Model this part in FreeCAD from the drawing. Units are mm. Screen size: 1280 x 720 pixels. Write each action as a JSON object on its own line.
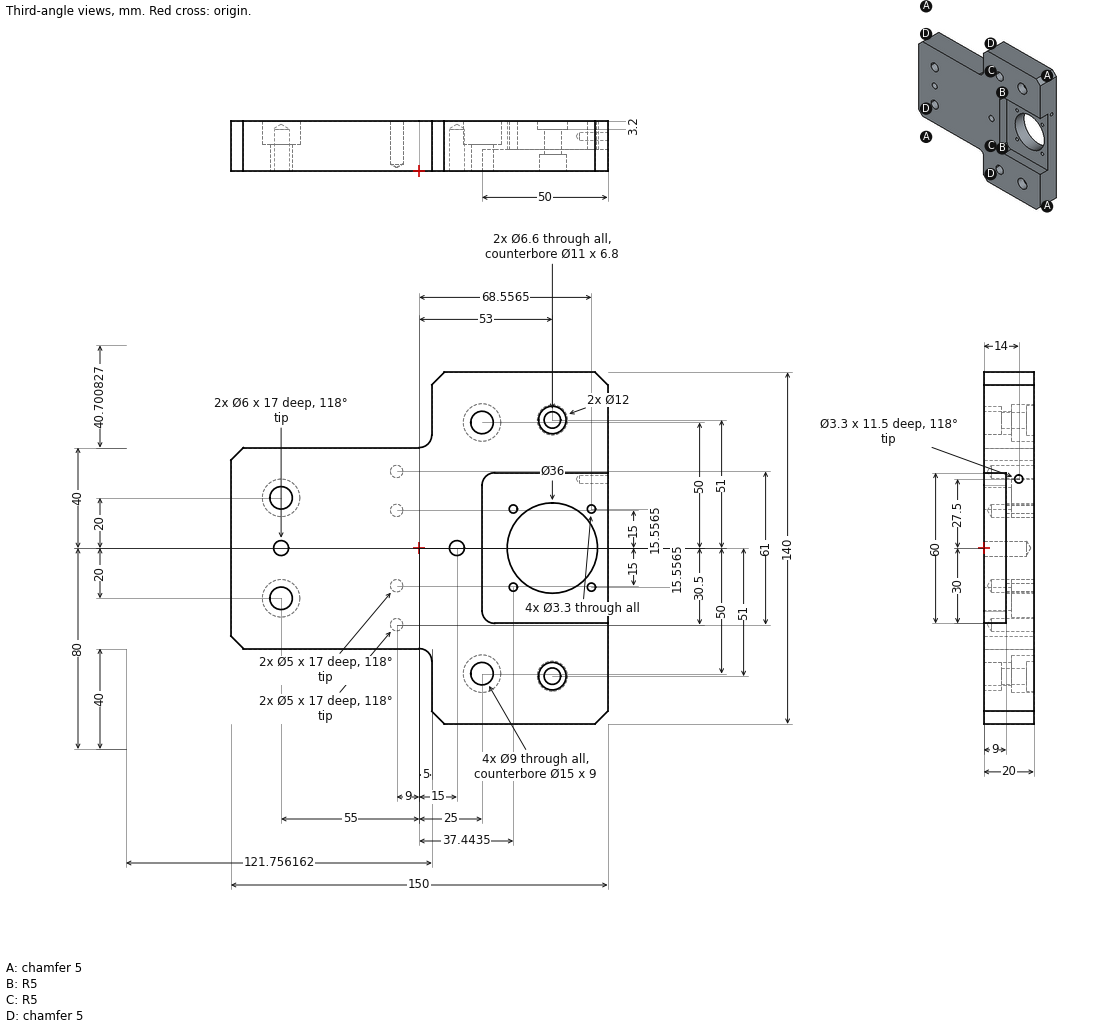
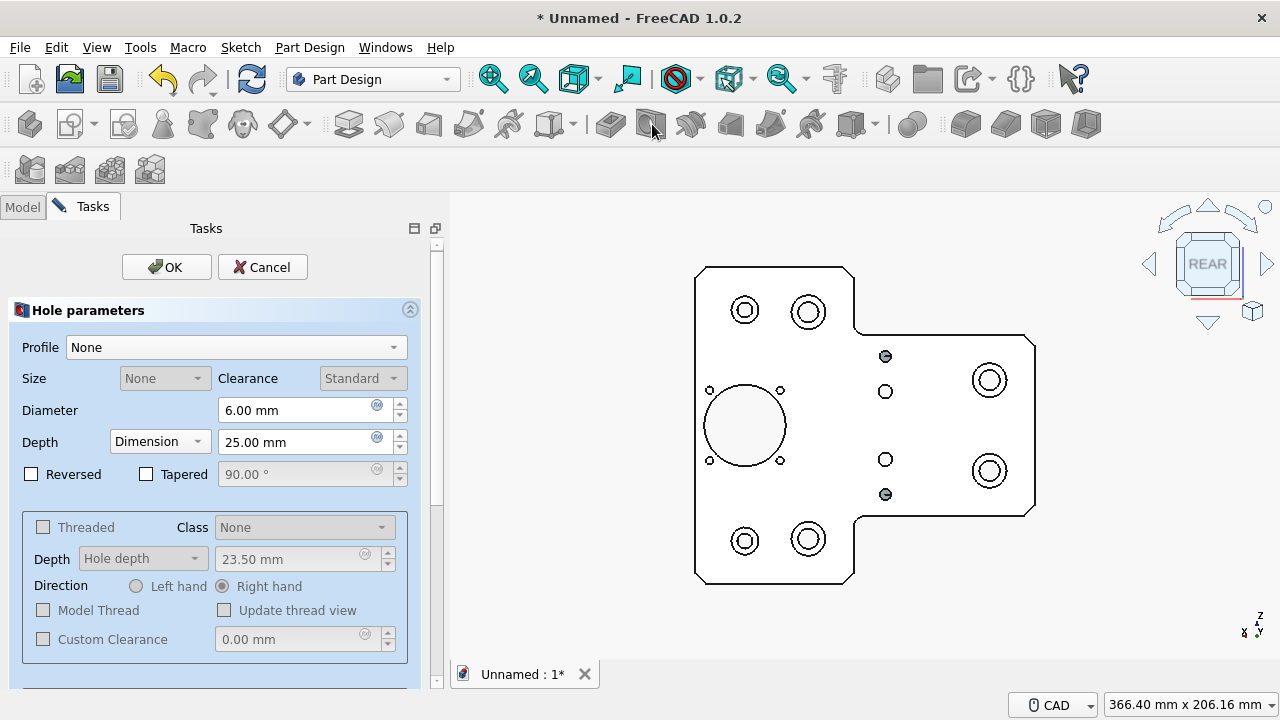
{"action": "triple_click", "coordinate": [305, 410]}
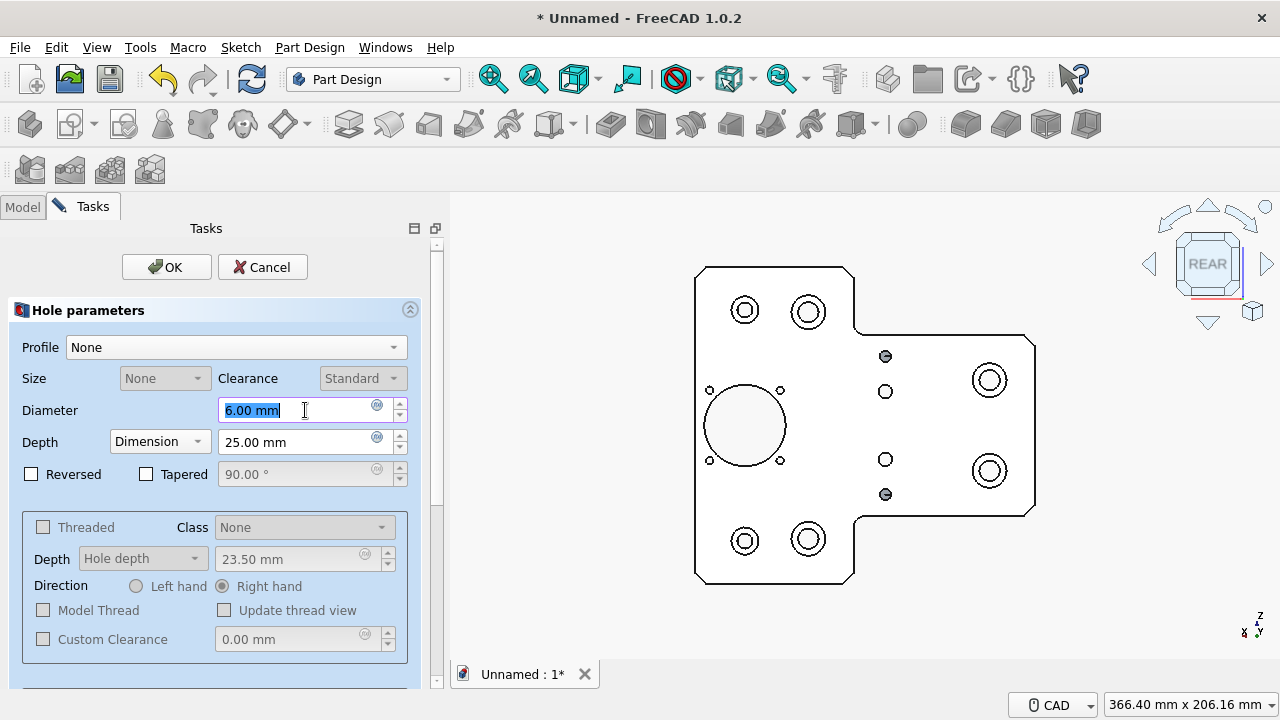
{"action": "type", "text": "5"}
{"action": "key", "text": "Tab"}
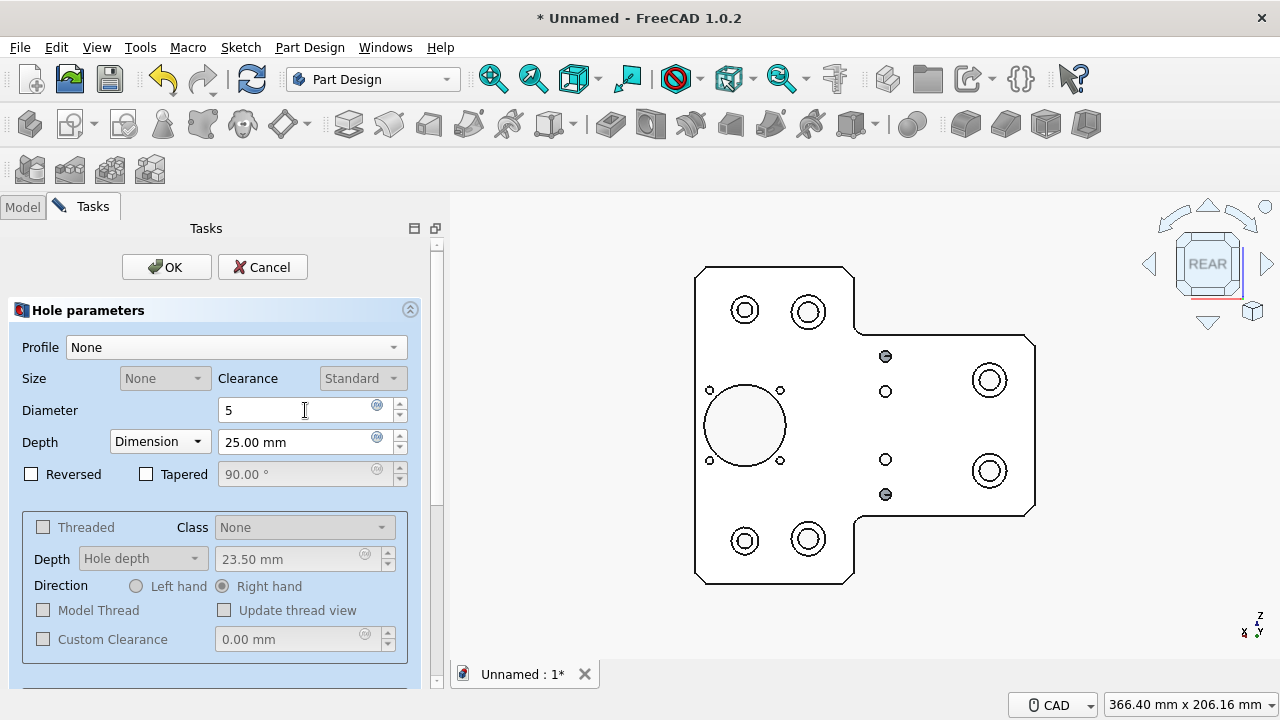
{"action": "triple_click", "coordinate": [305, 442]}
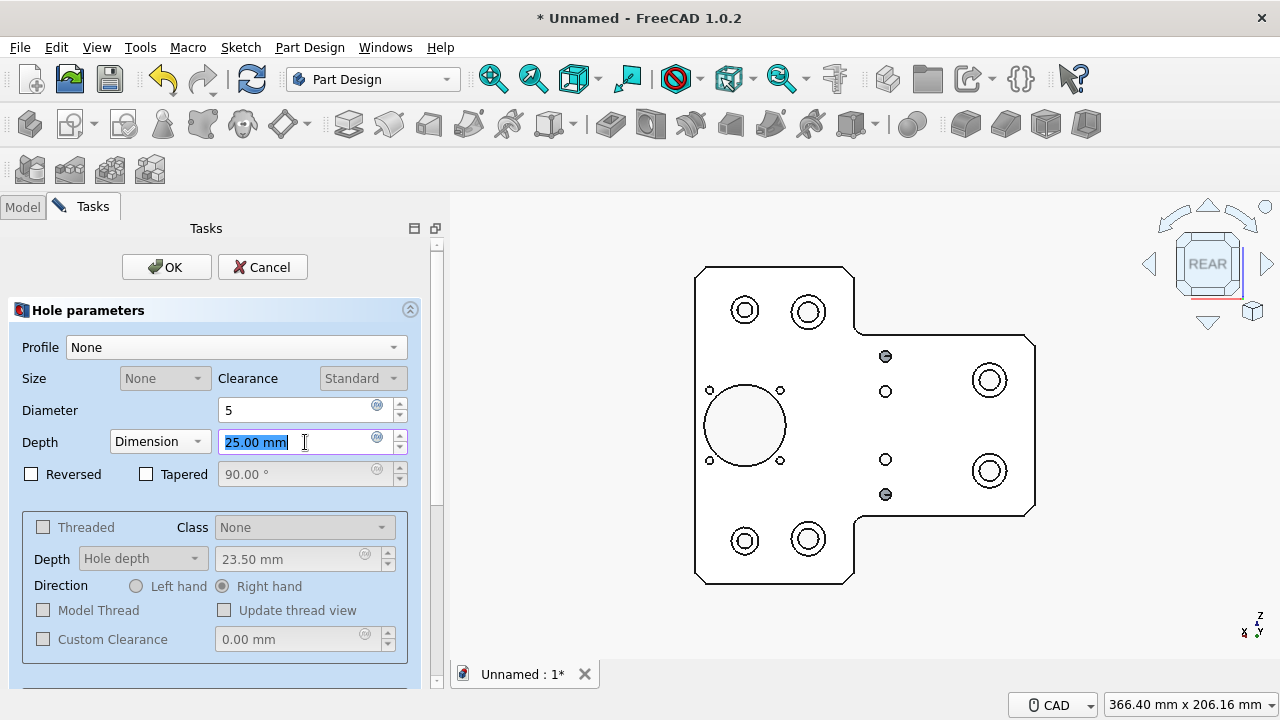
{"action": "type", "text": "17"}
{"action": "key", "text": "Tab"}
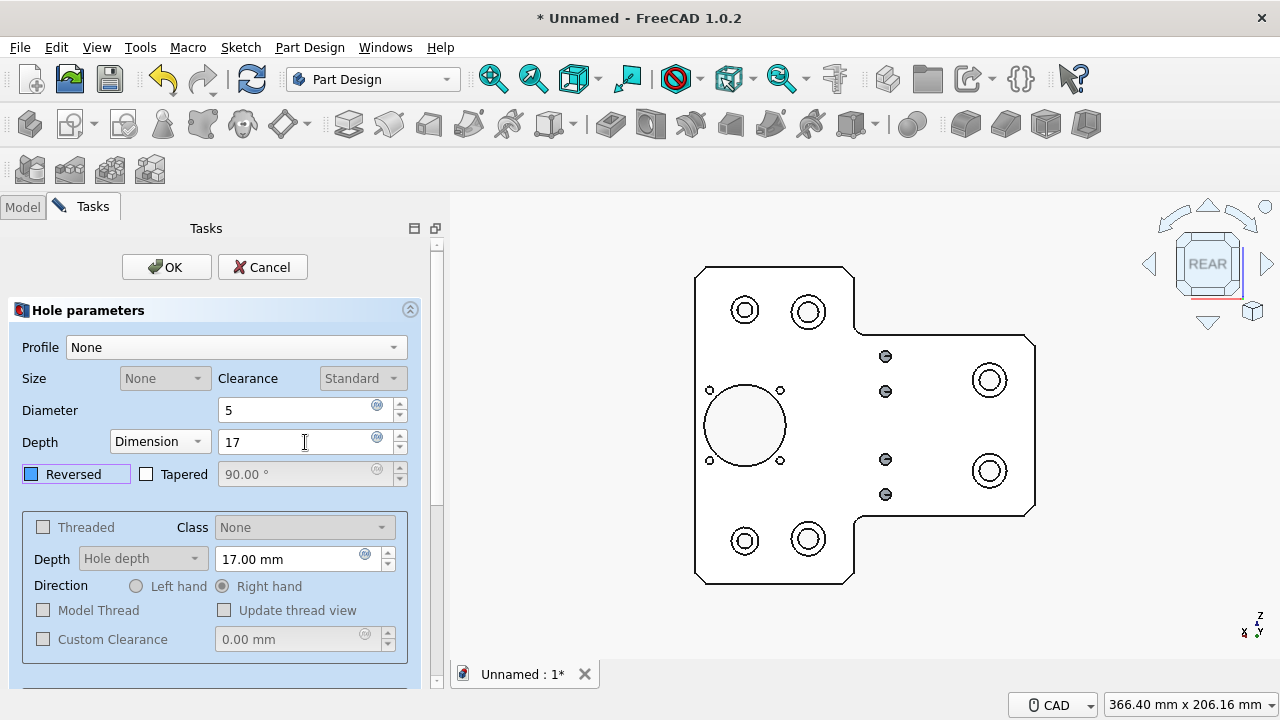
{"action": "left_click", "coordinate": [167, 267]}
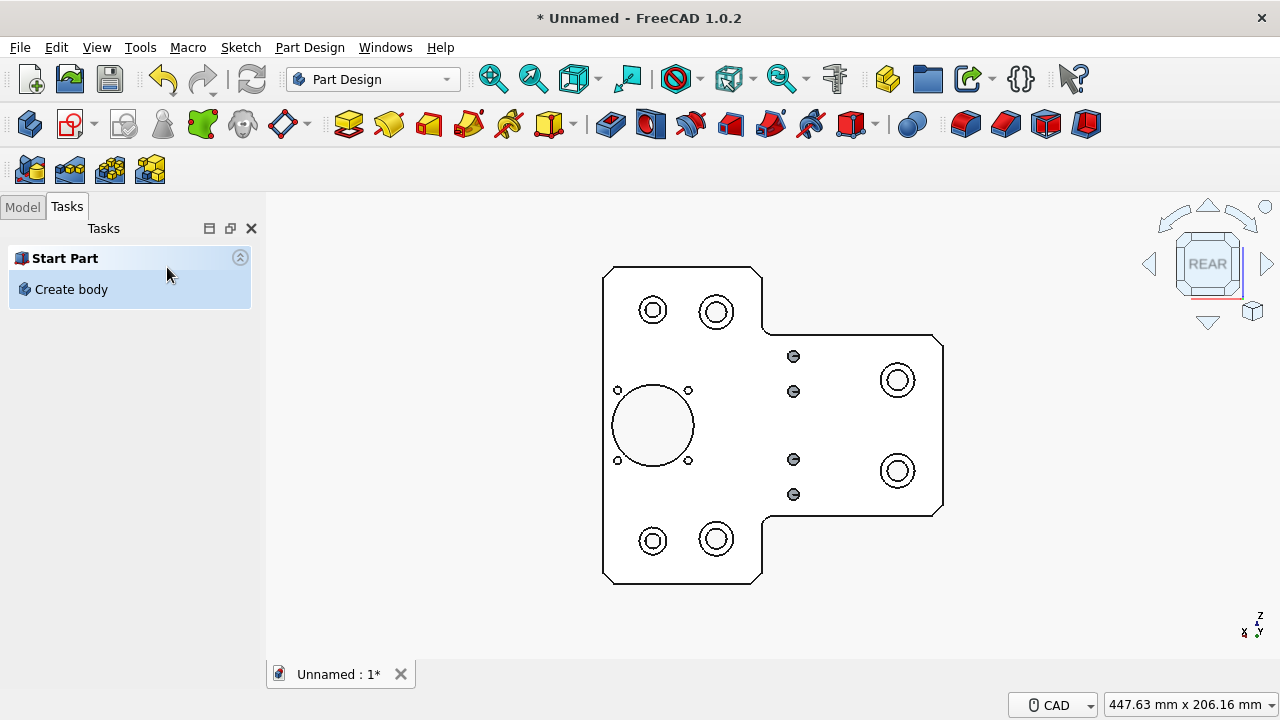
{"action": "key", "text": "0"}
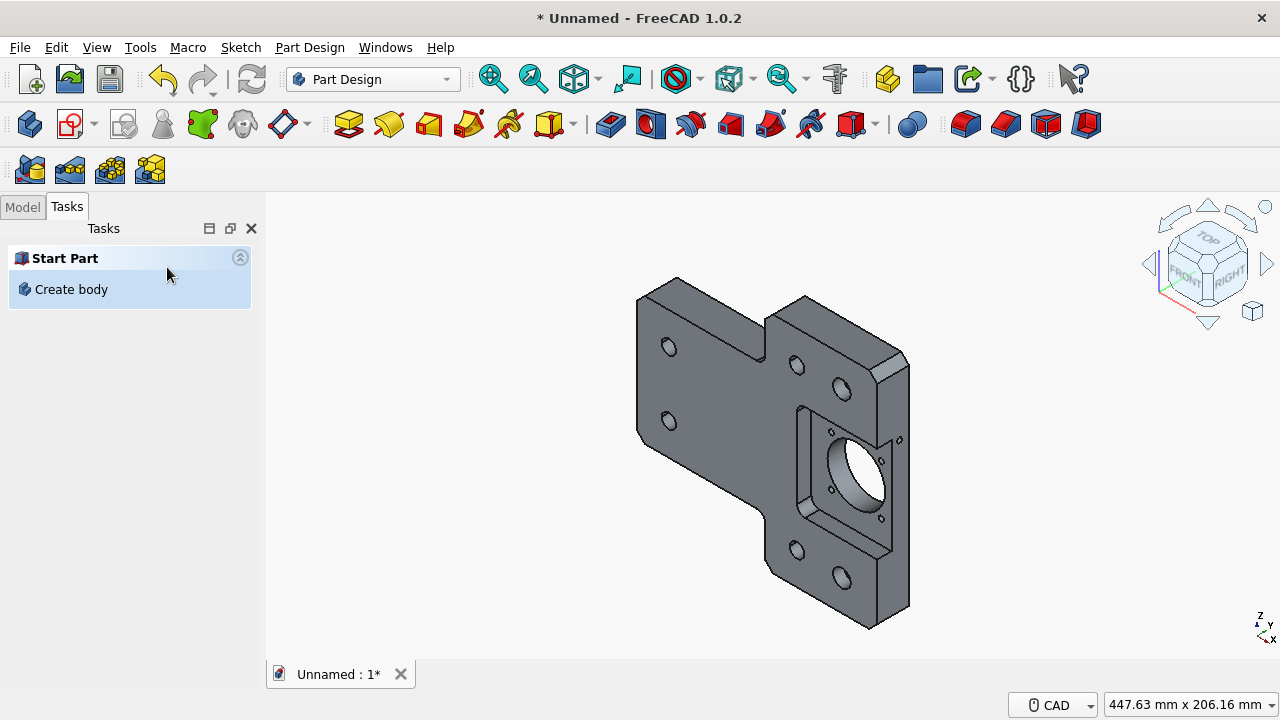
{"action": "left_click", "coordinate": [723, 414]}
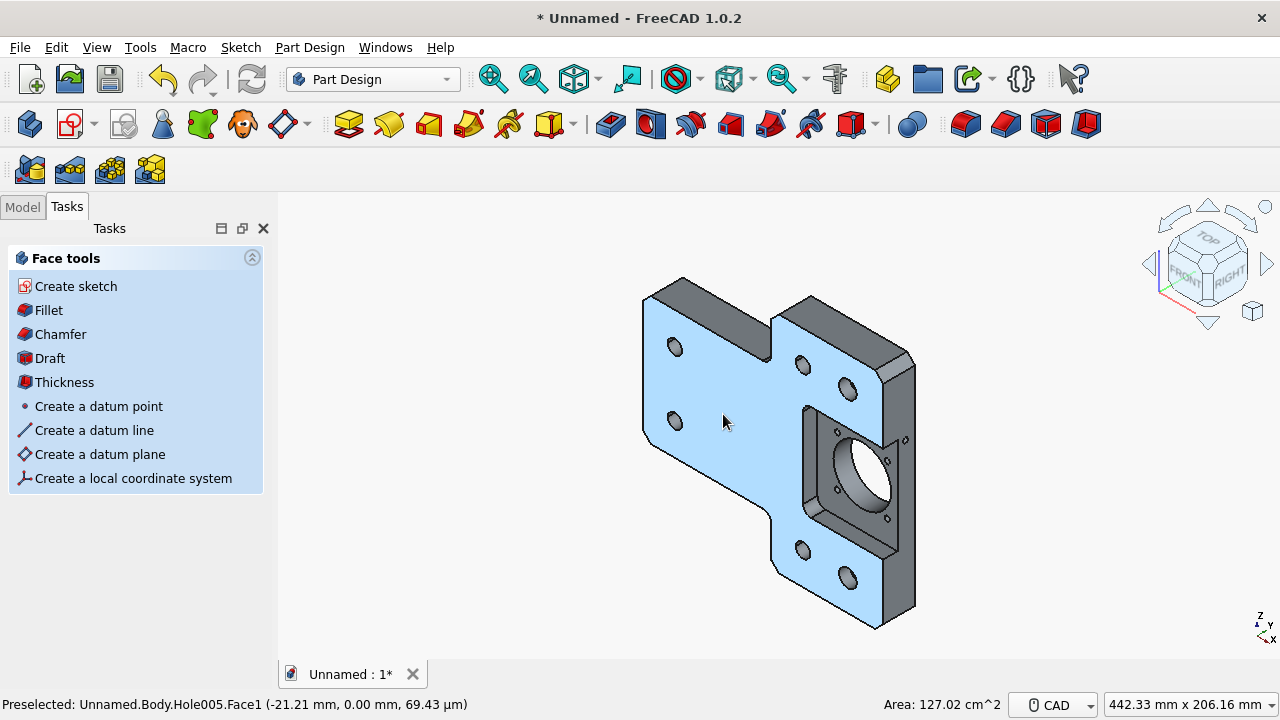
{"action": "left_click", "coordinate": [70, 124]}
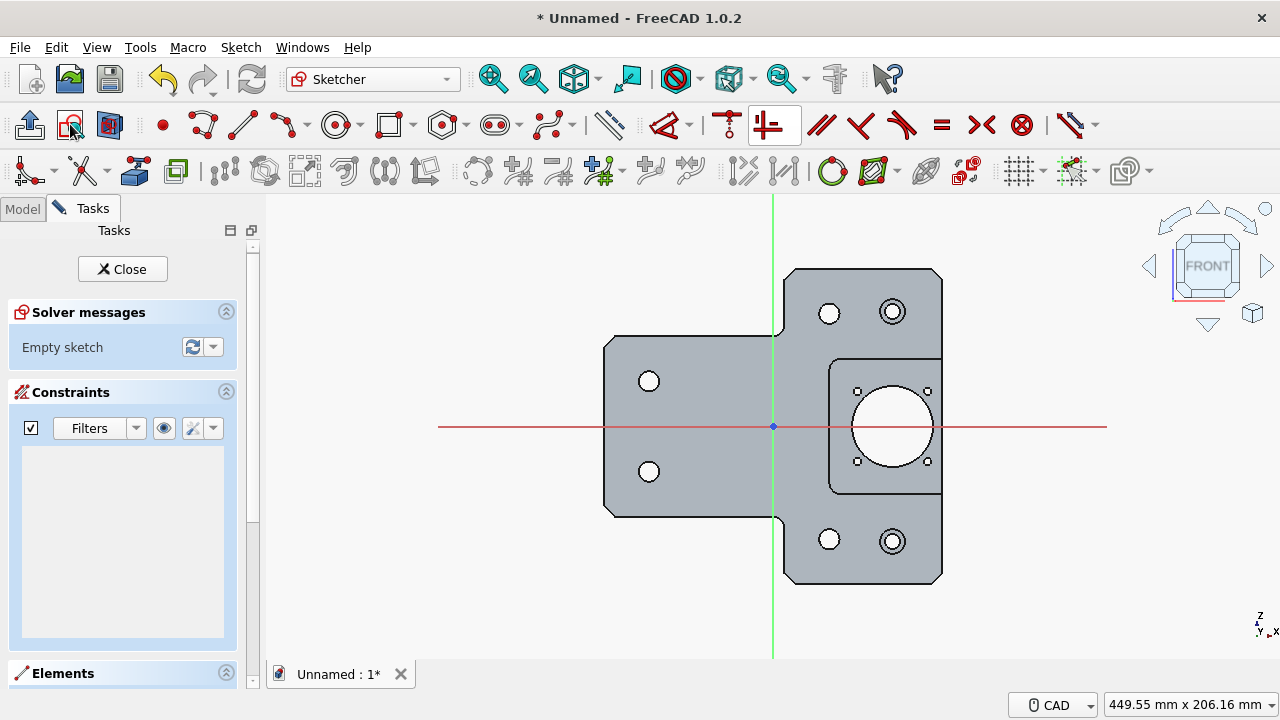
{"action": "scroll", "coordinate": [738, 427], "scroll_direction": "up", "scroll_amount": 6}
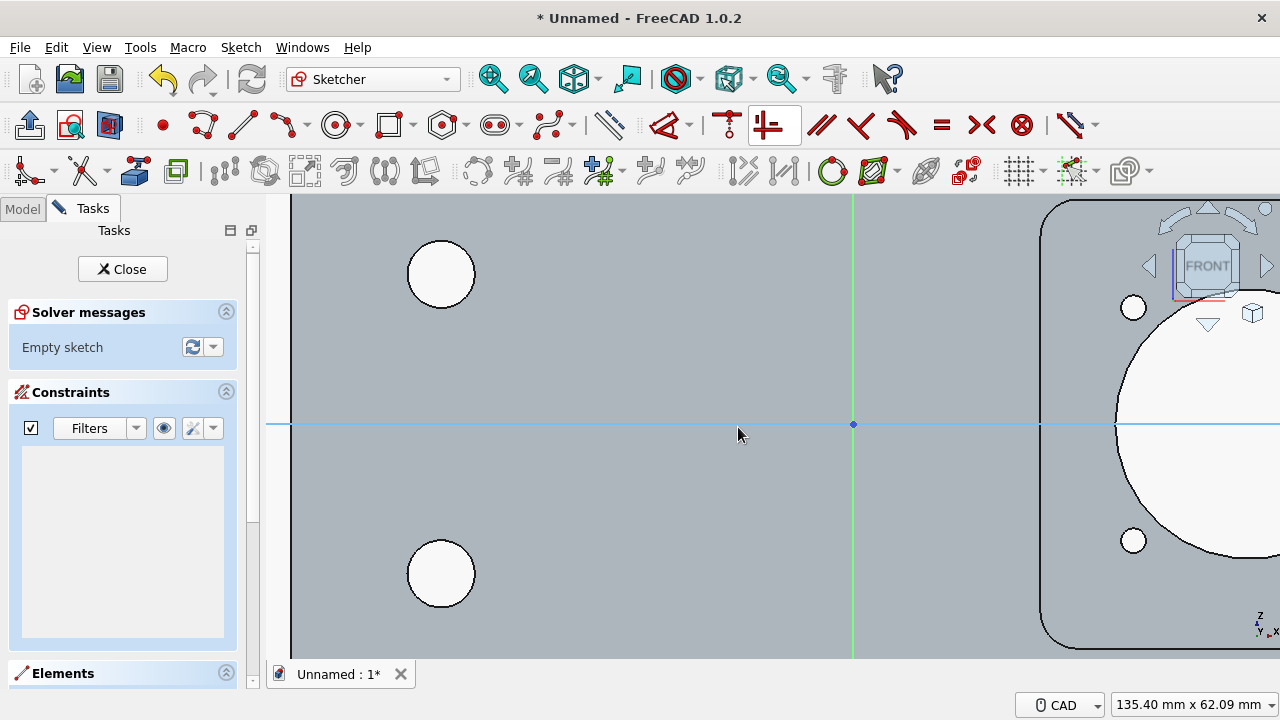
{"action": "left_click", "coordinate": [336, 126]}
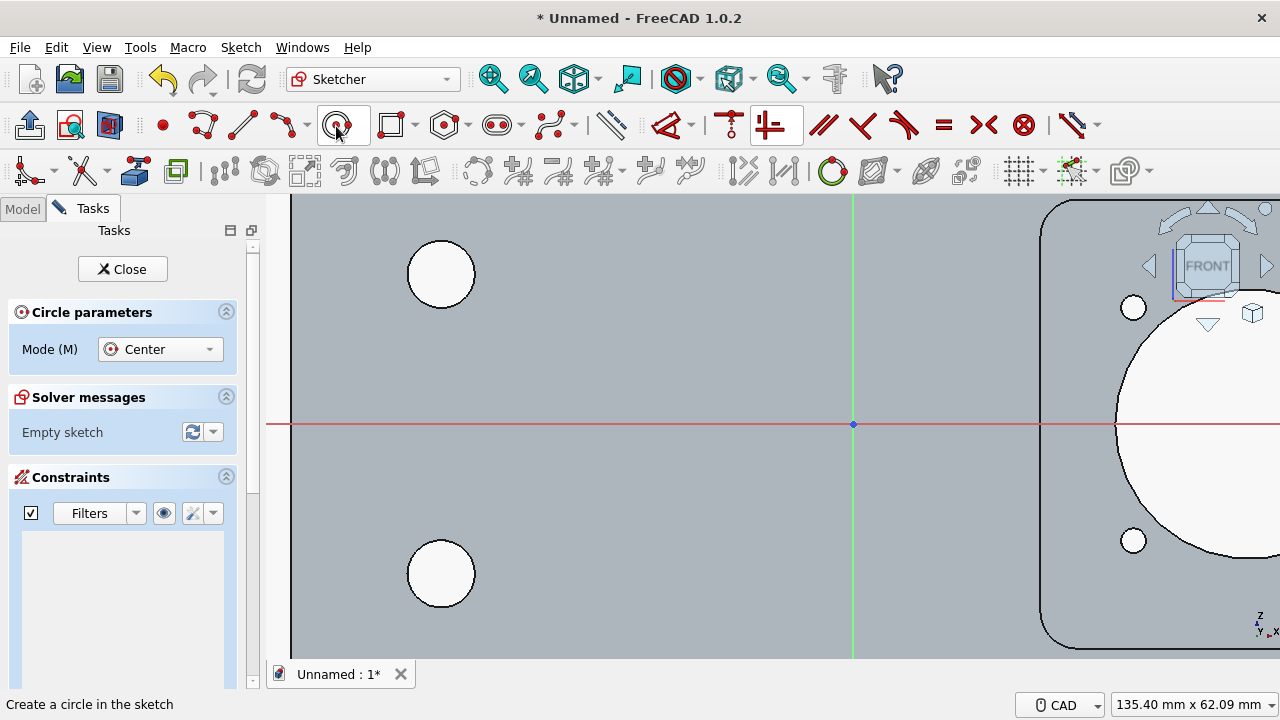
{"action": "left_click", "coordinate": [441, 424]}
{"action": "left_click", "coordinate": [457, 408]}